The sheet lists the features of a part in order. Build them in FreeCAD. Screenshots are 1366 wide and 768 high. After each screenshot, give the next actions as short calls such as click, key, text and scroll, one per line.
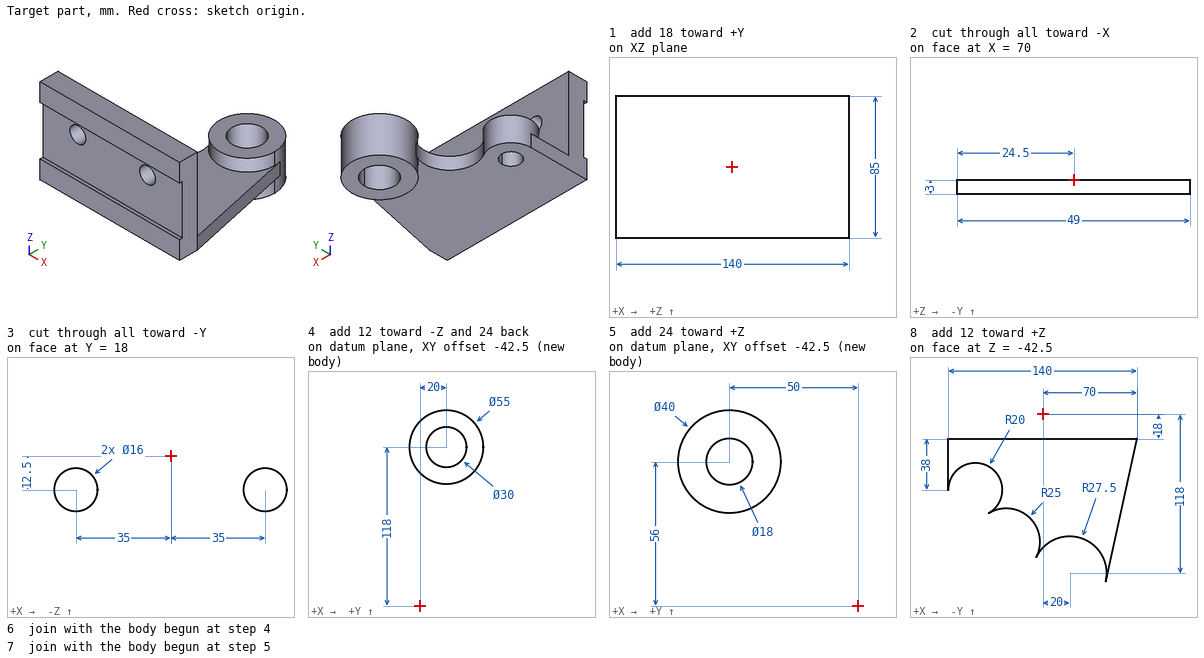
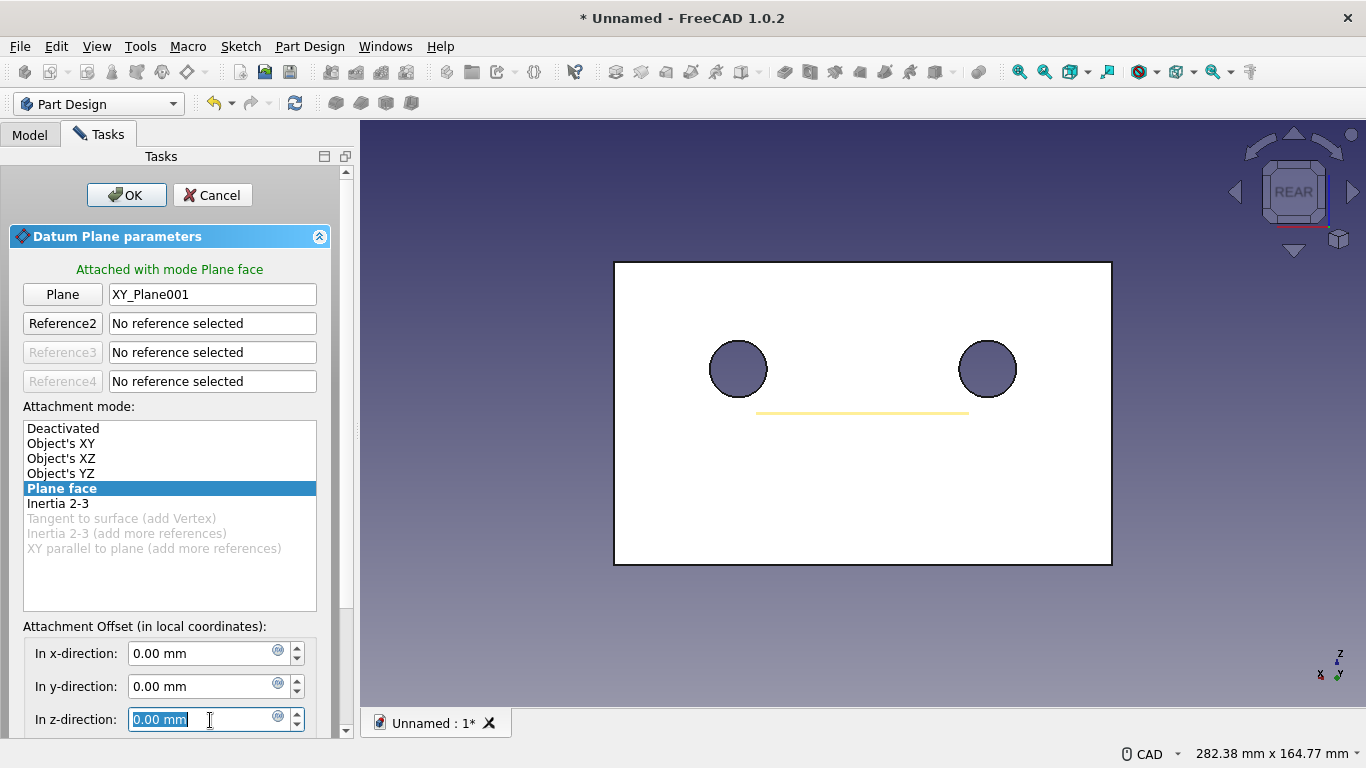
text(-42.5)
key(Tab)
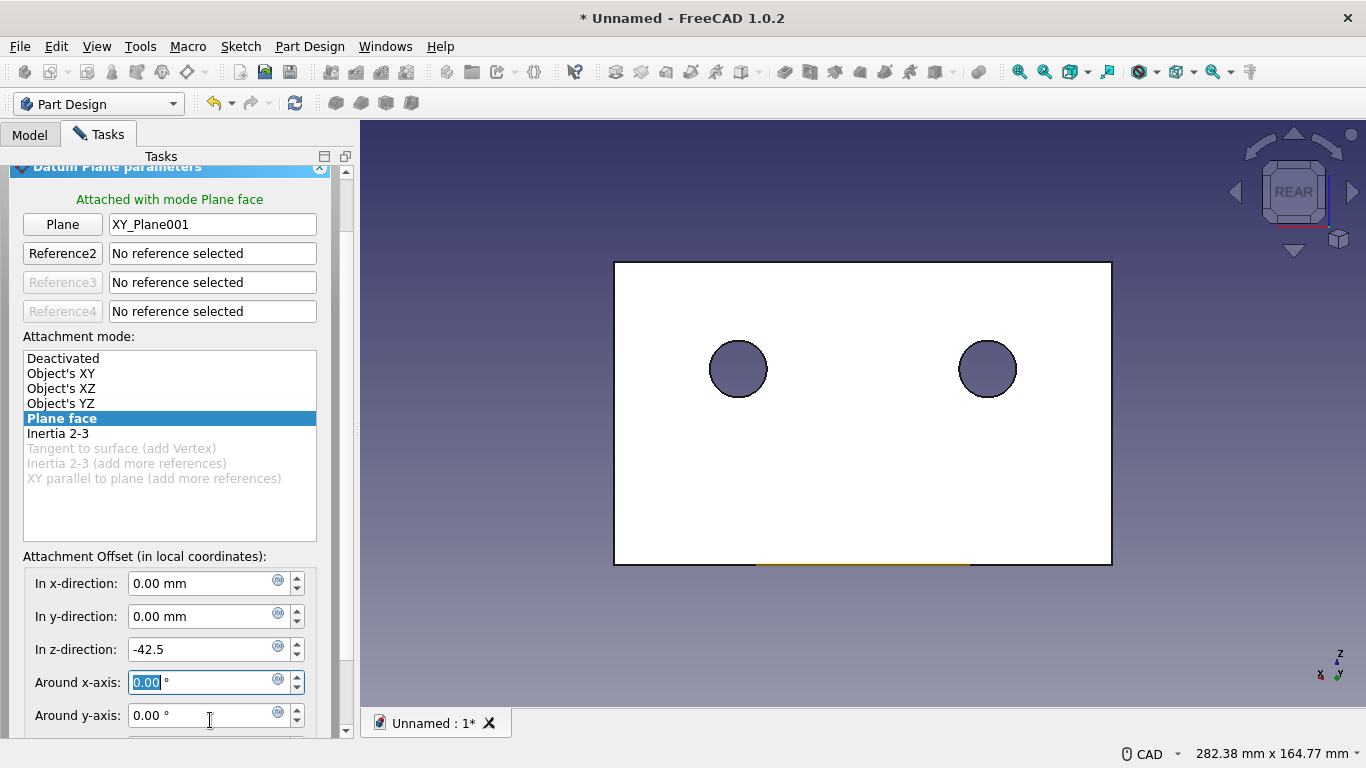
scroll(346, 452, up, 2)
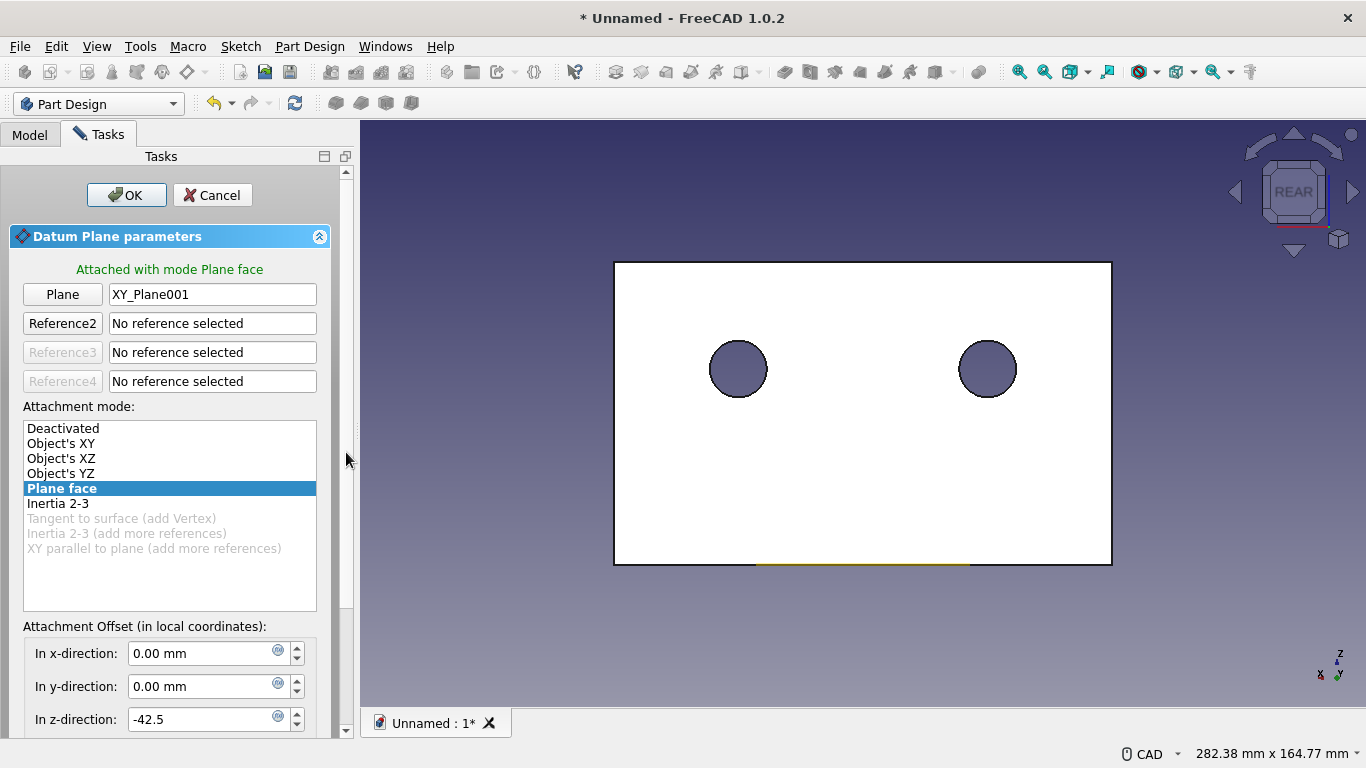
click(127, 195)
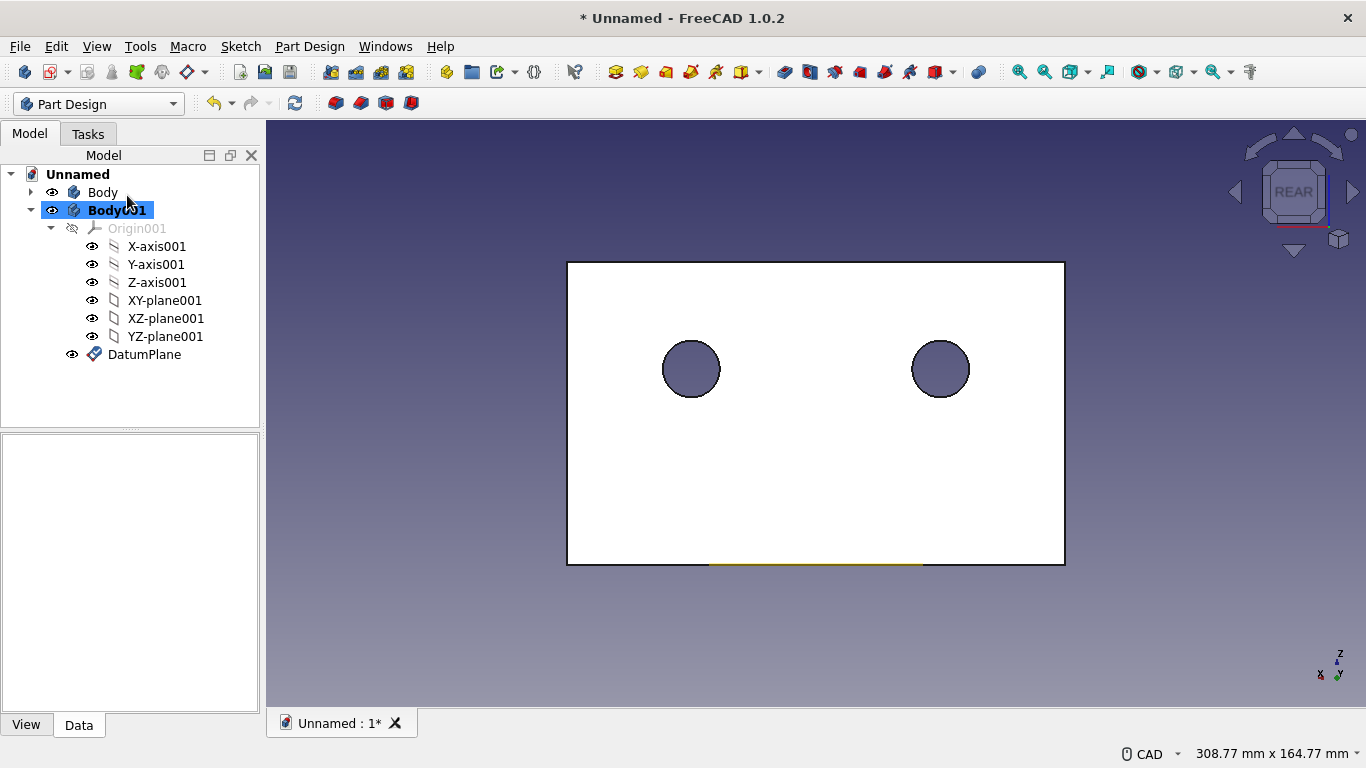
click(117, 354)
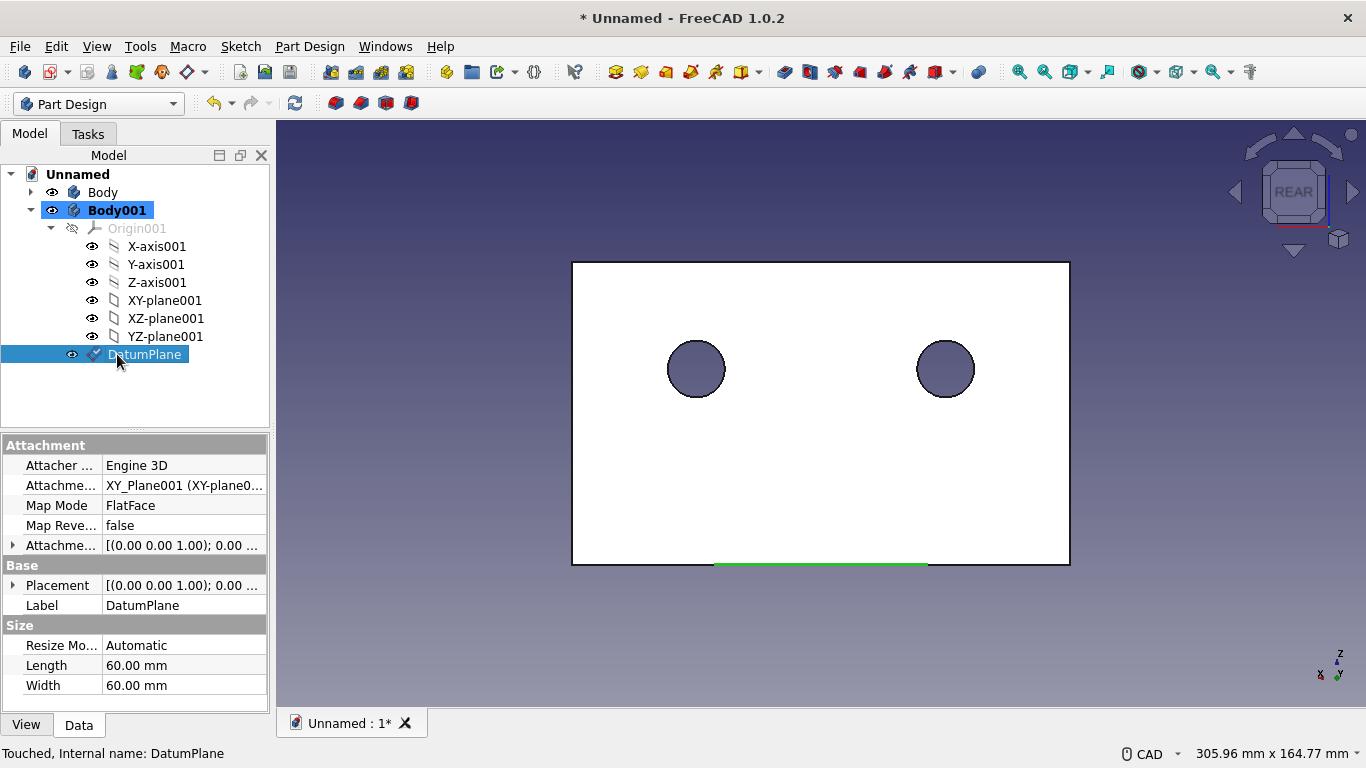
click(50, 72)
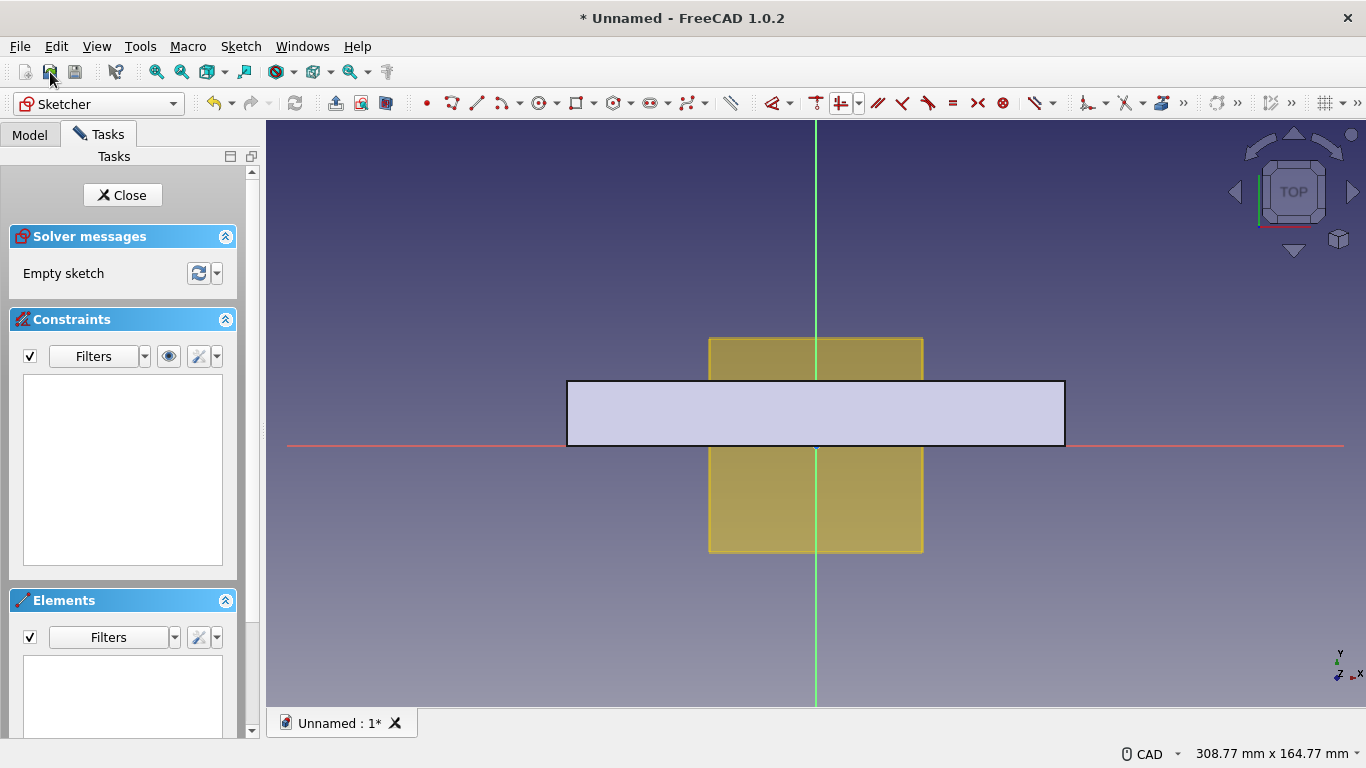
scroll(748, 414, down, 5)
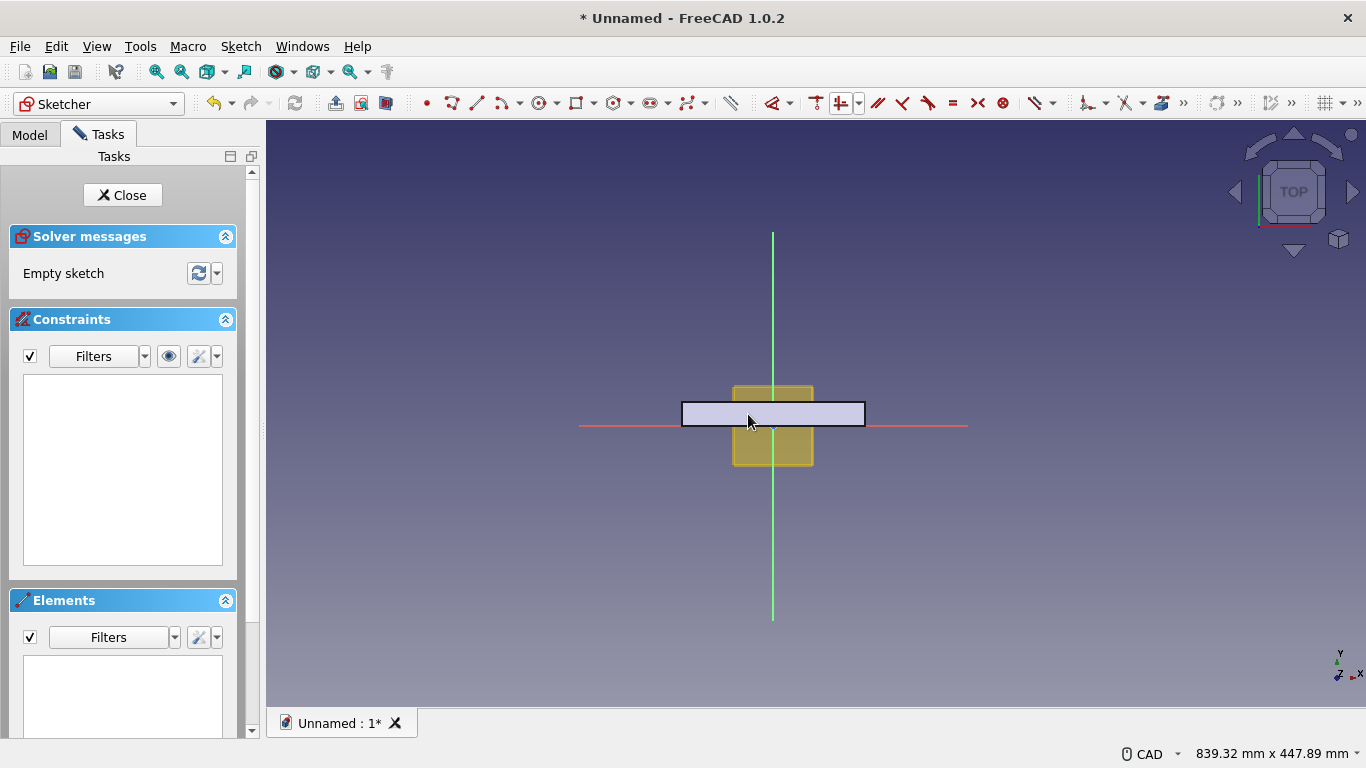
scroll(813, 235, up, 8)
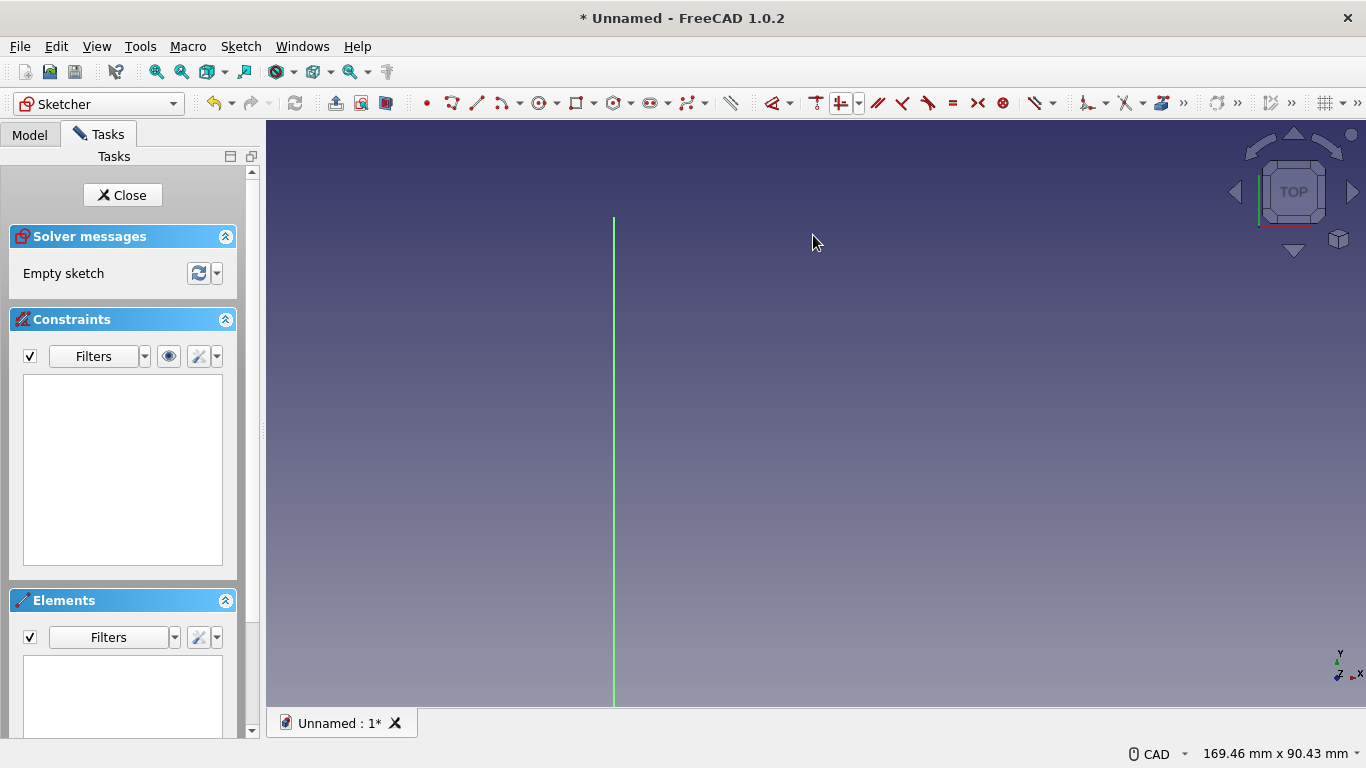
click(538, 104)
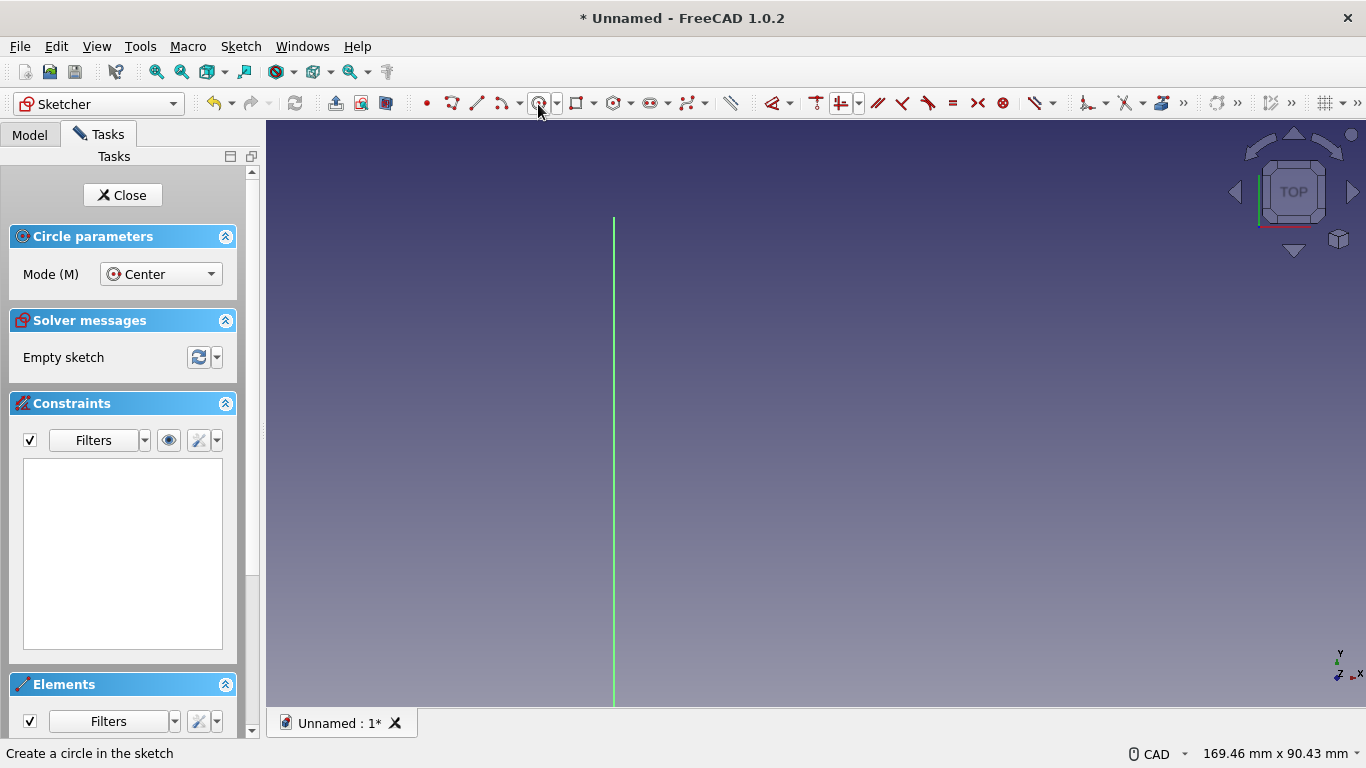
click(744, 414)
click(870, 288)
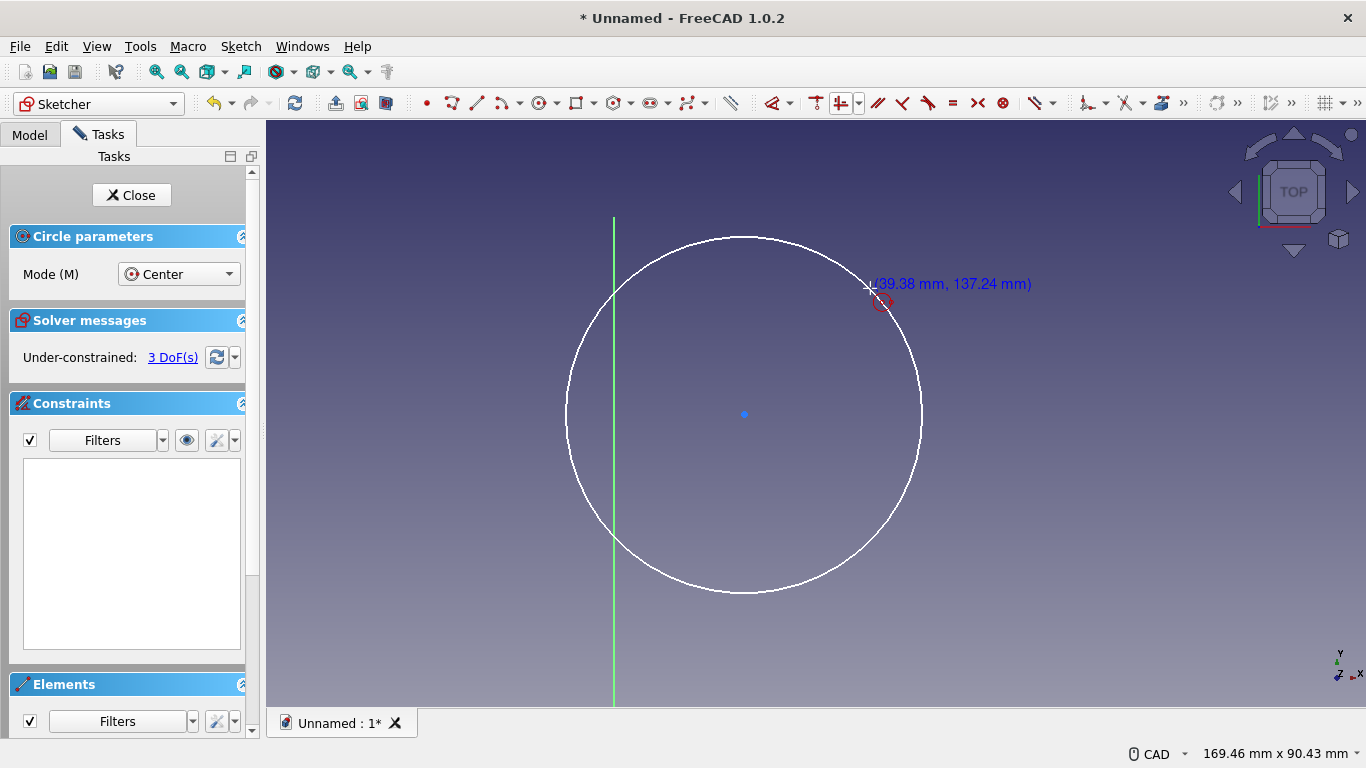
click(744, 415)
click(813, 345)
key(Escape)